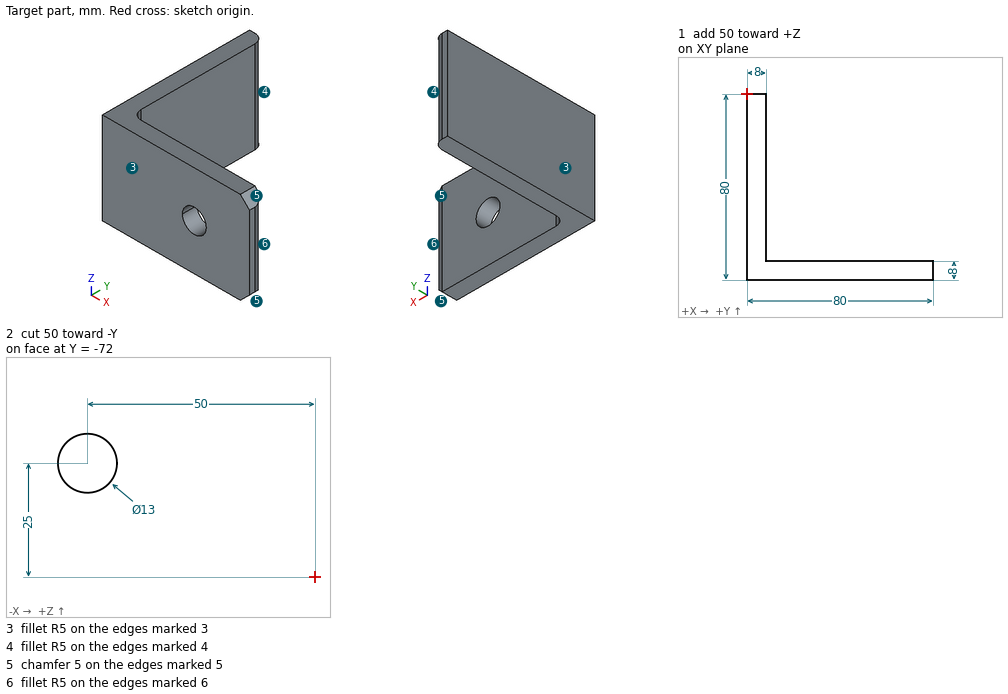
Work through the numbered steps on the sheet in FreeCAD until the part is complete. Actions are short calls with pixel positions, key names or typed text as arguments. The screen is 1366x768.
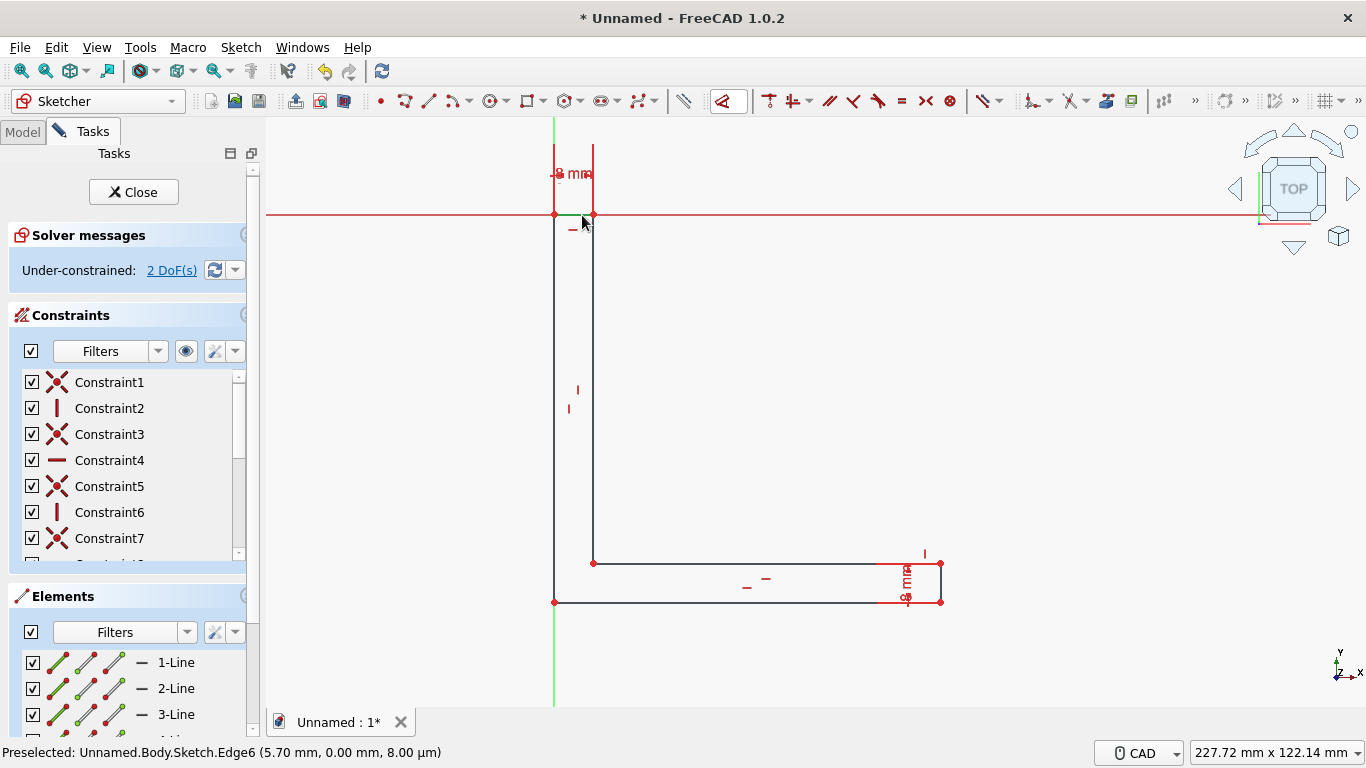
click(554, 331)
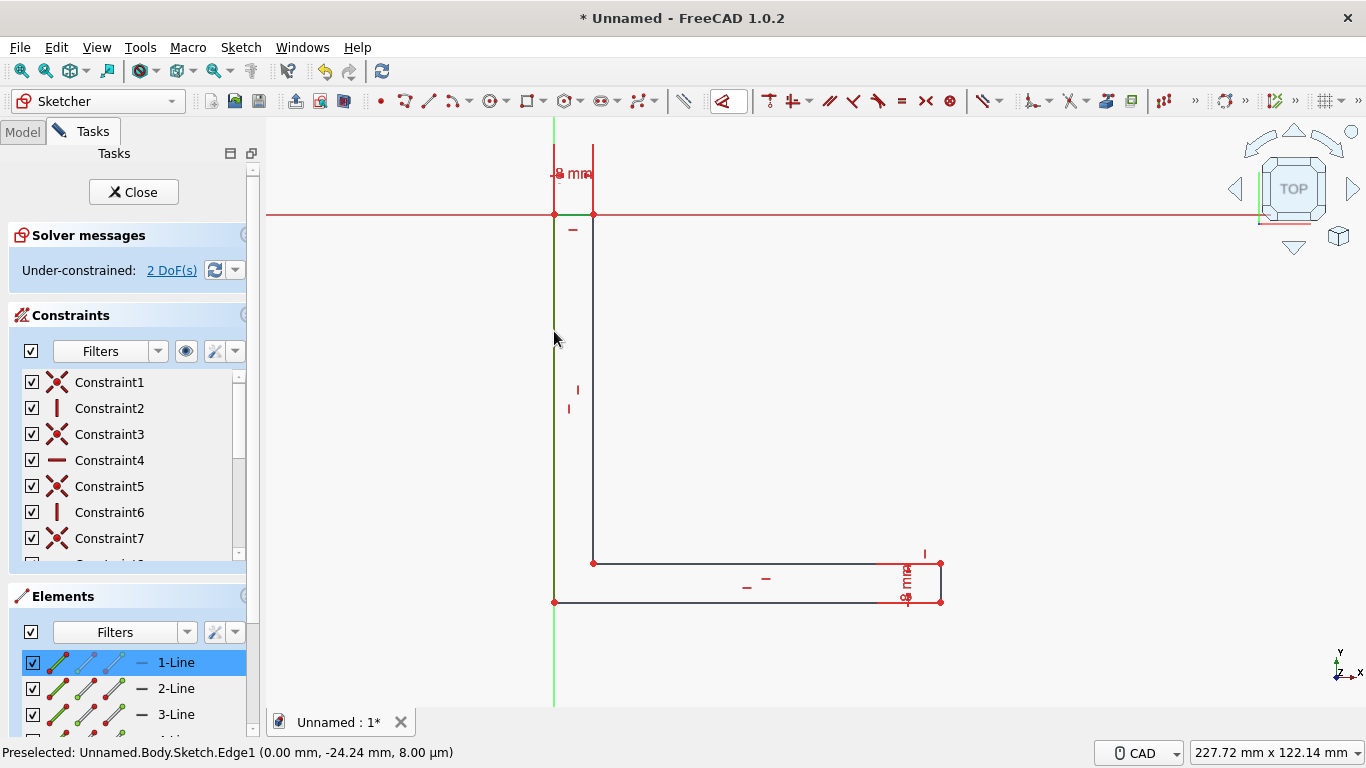
click(742, 102)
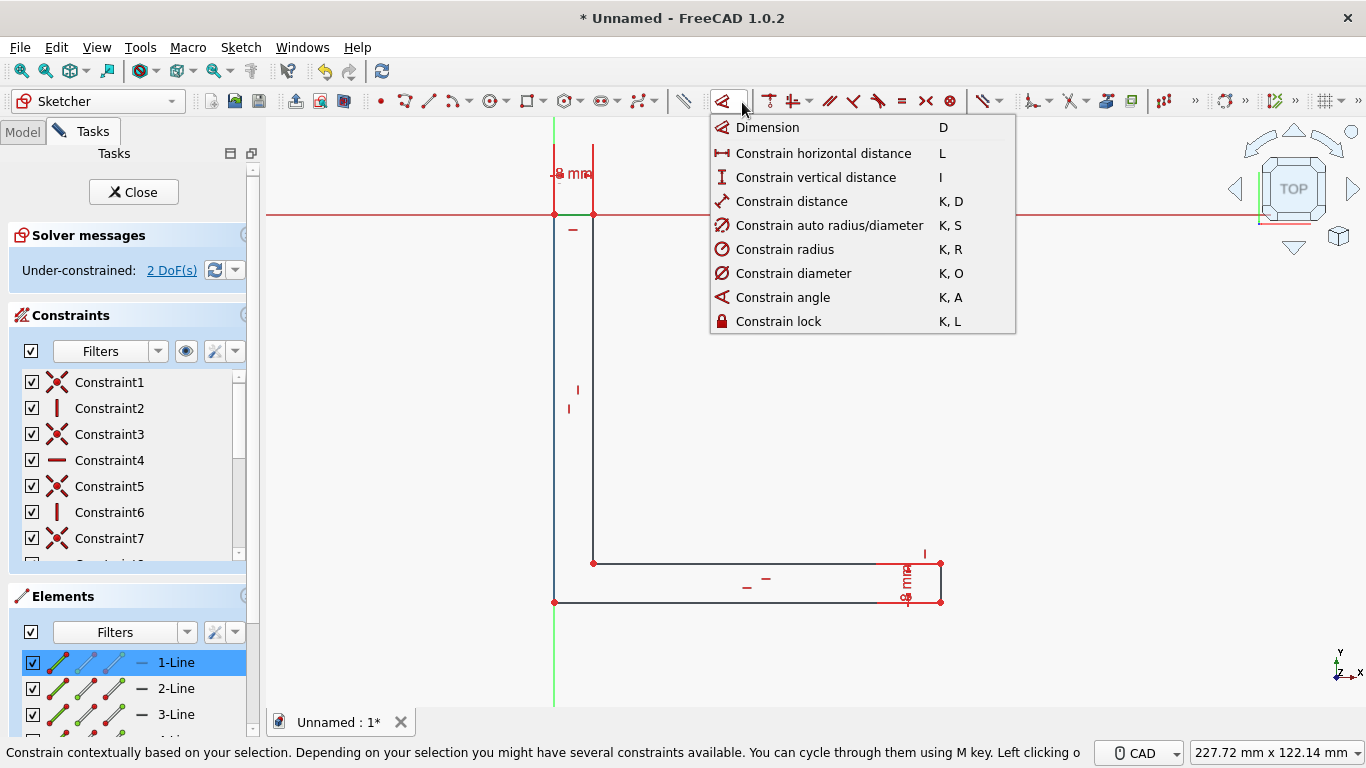
click(863, 177)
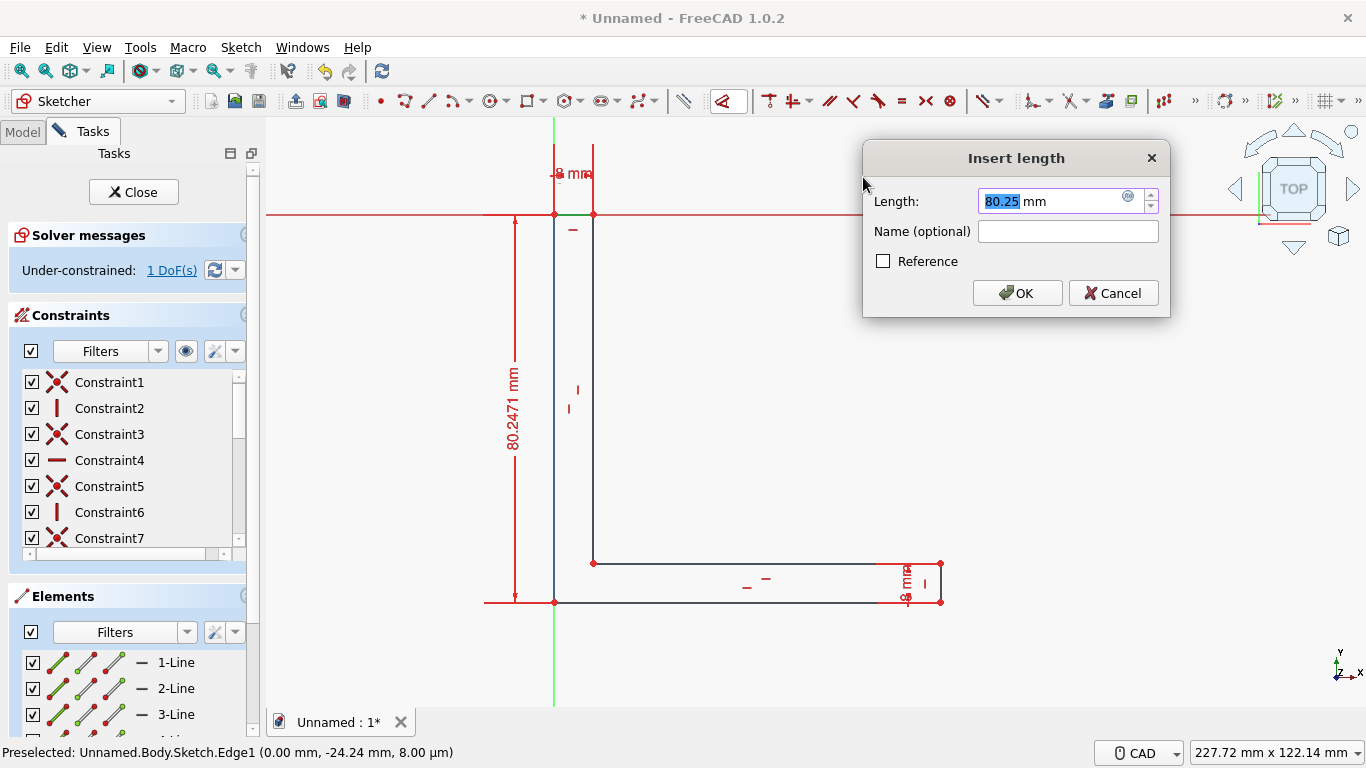
text(80)
key(Return)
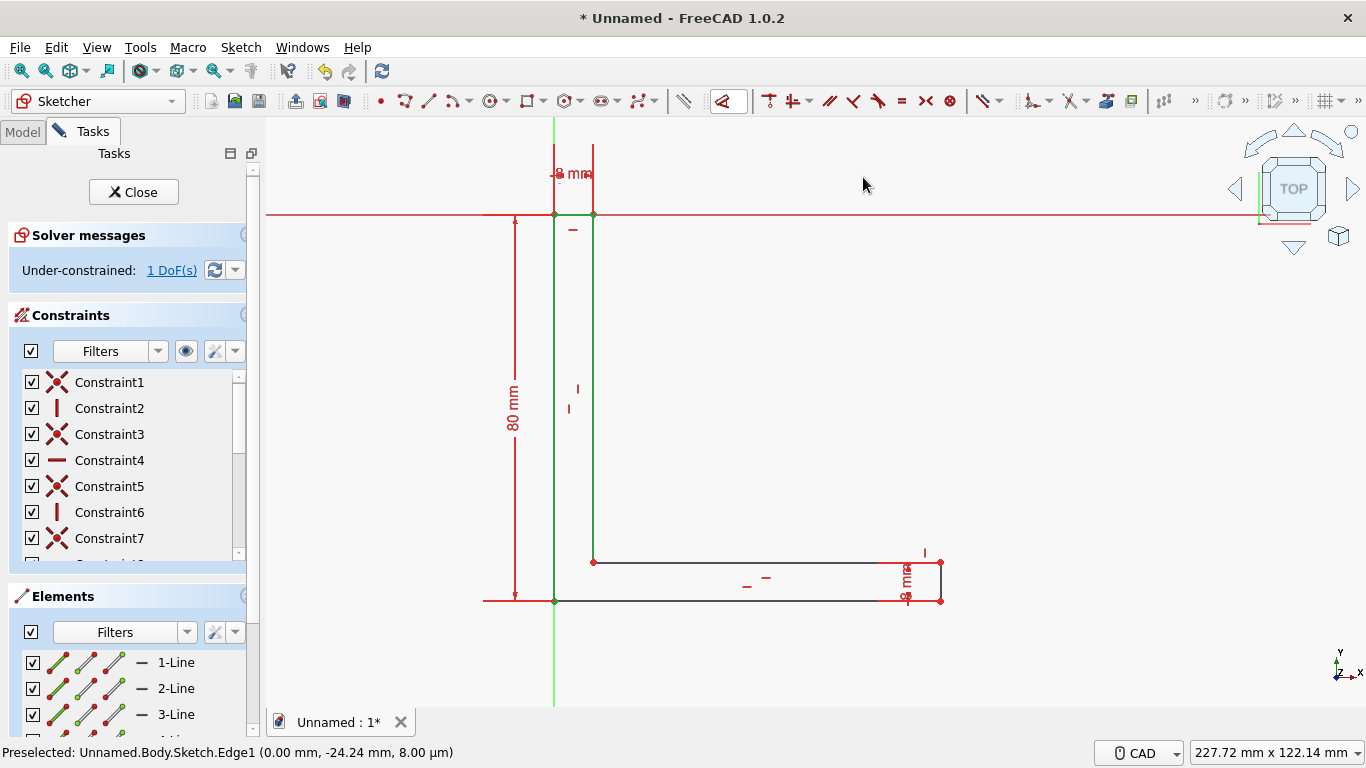
click(670, 601)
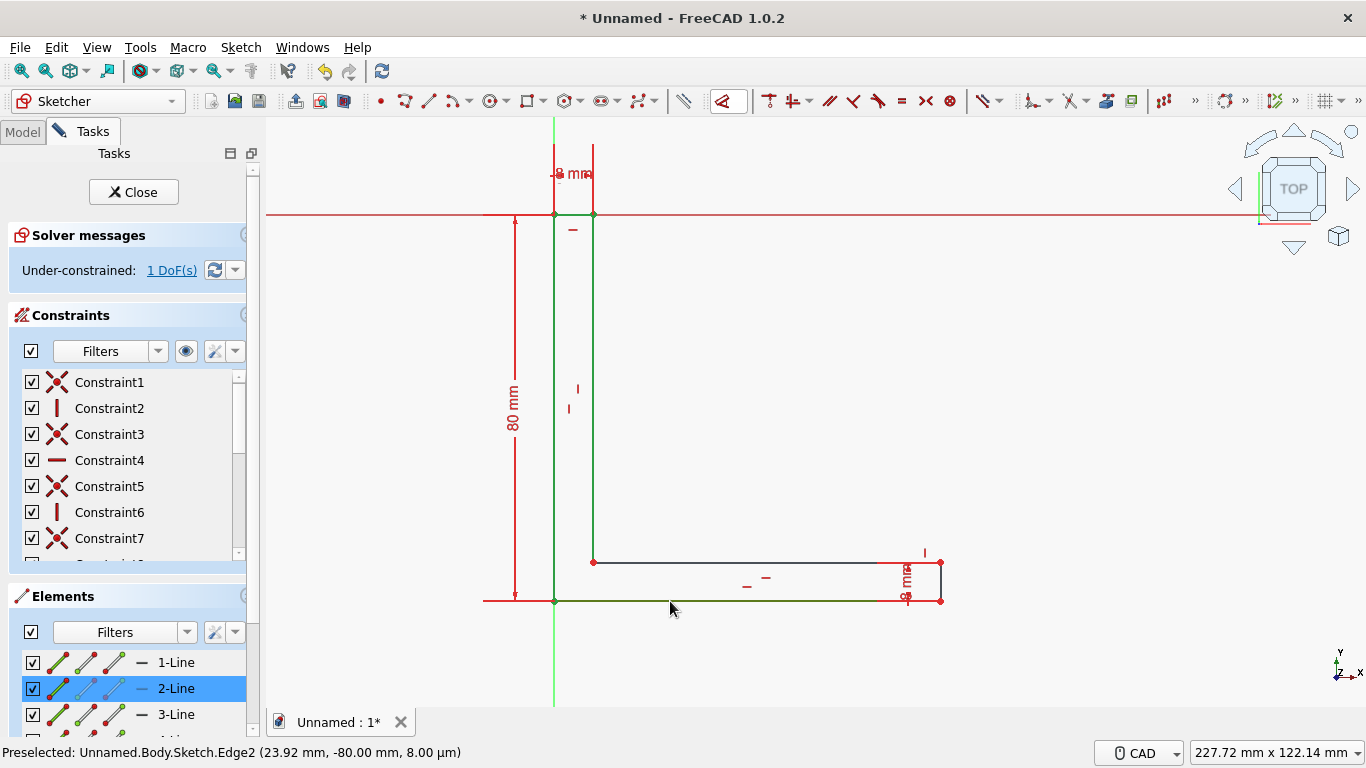
key(l)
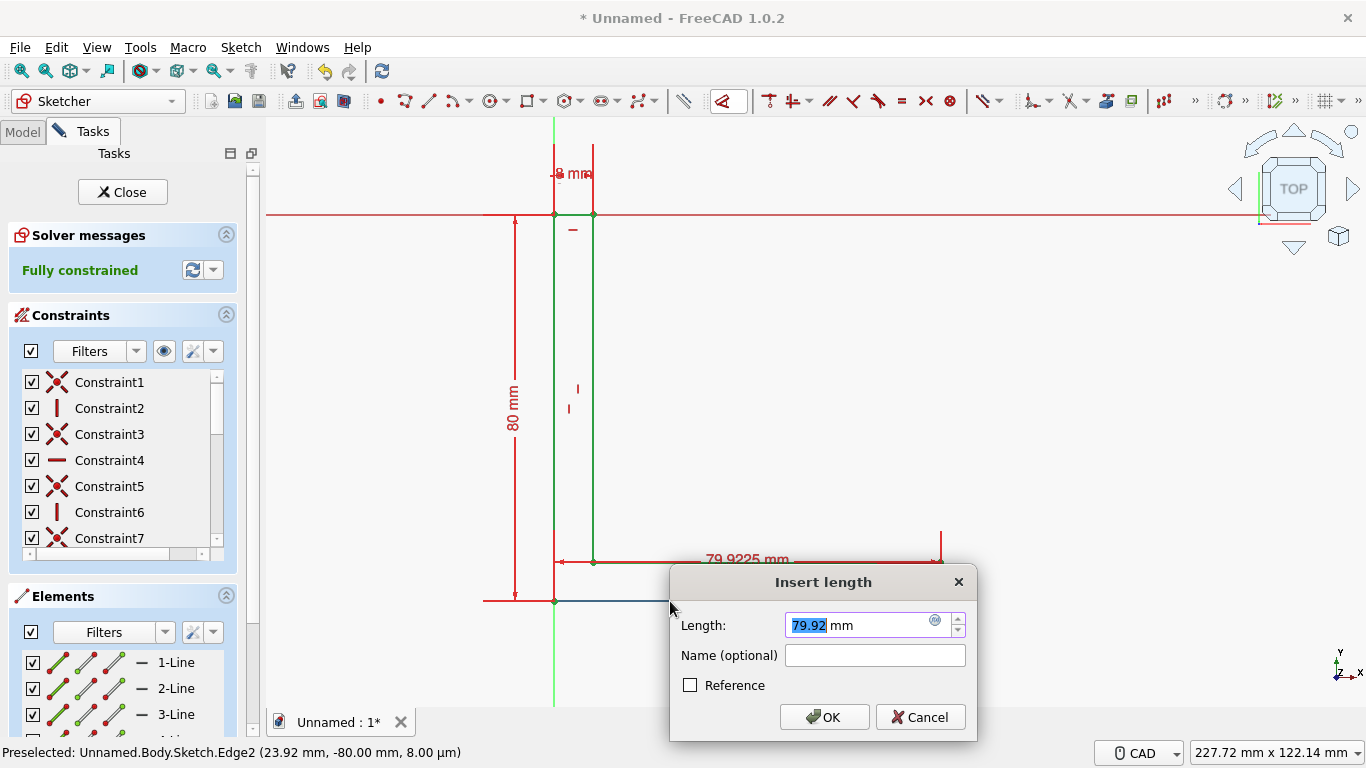
text(80)
key(Return)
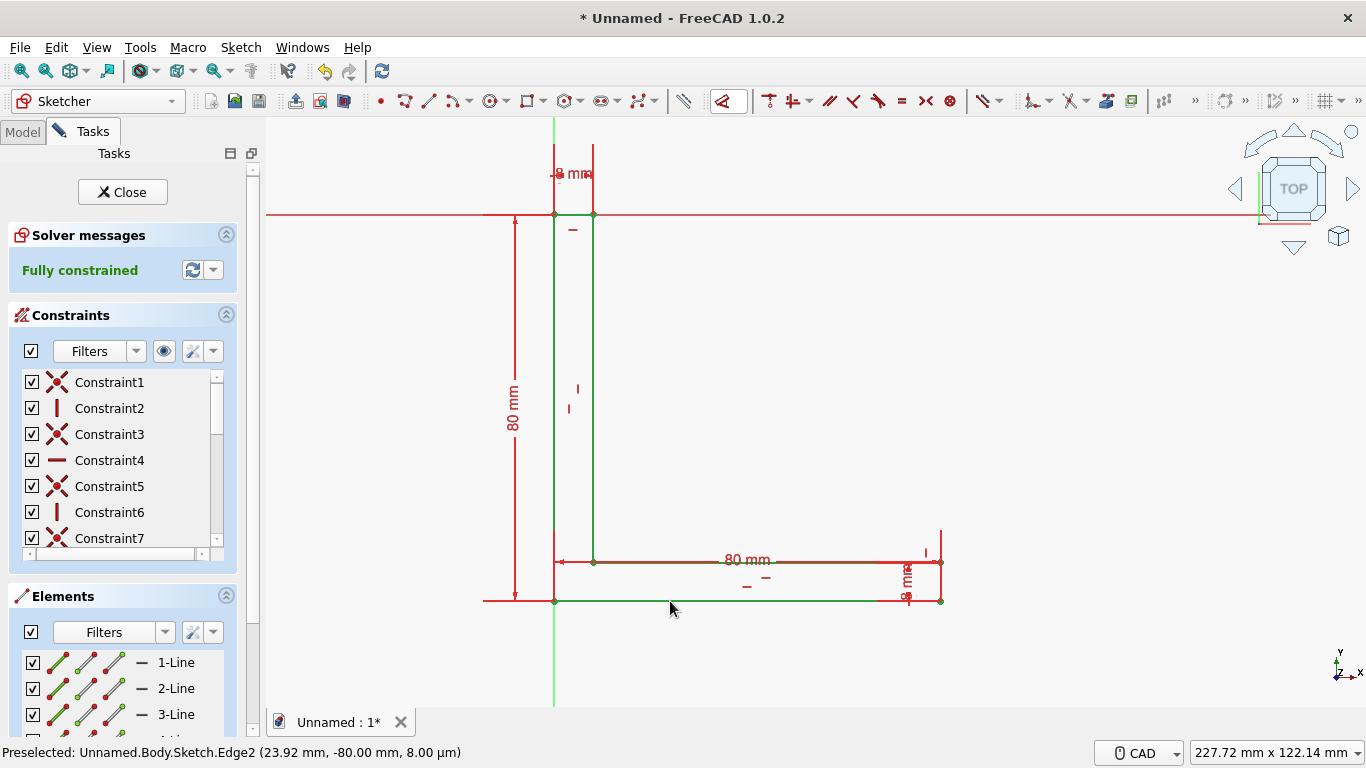
click(123, 192)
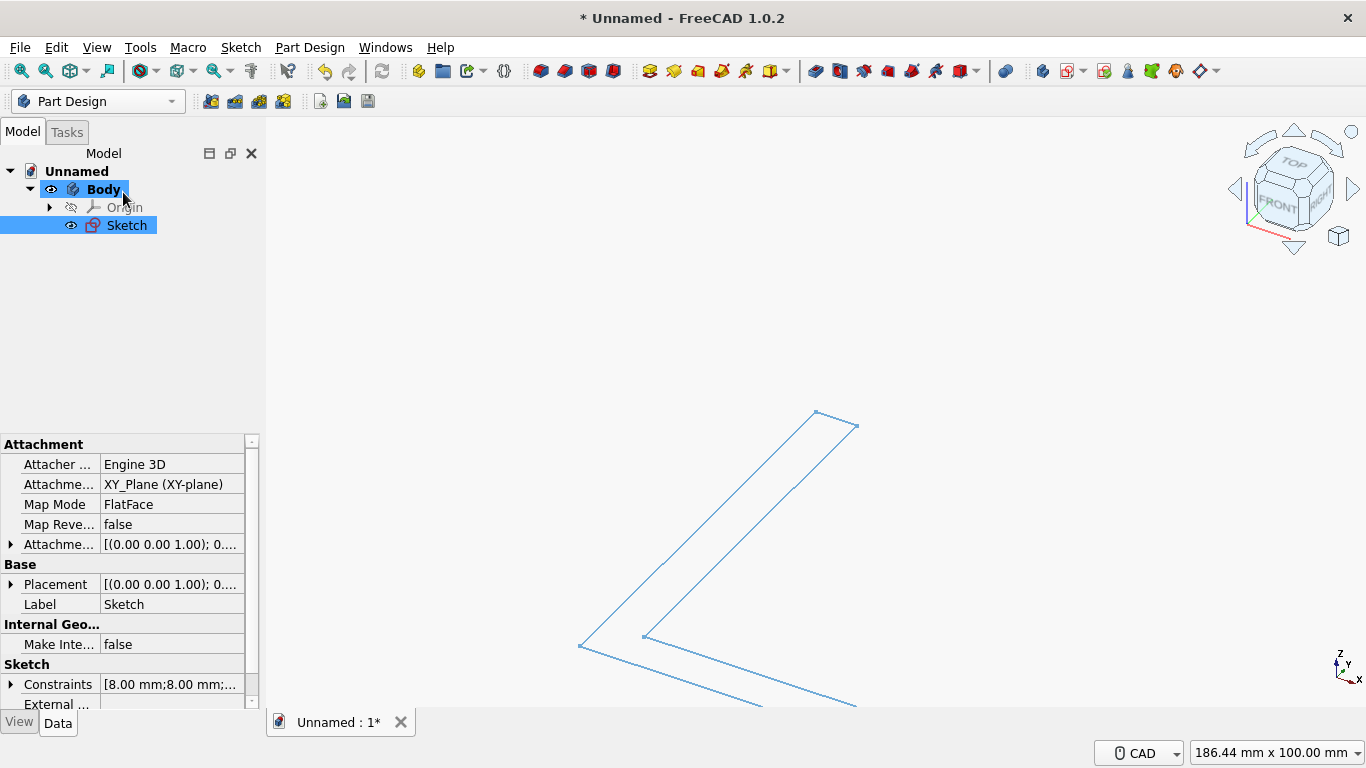
click(650, 72)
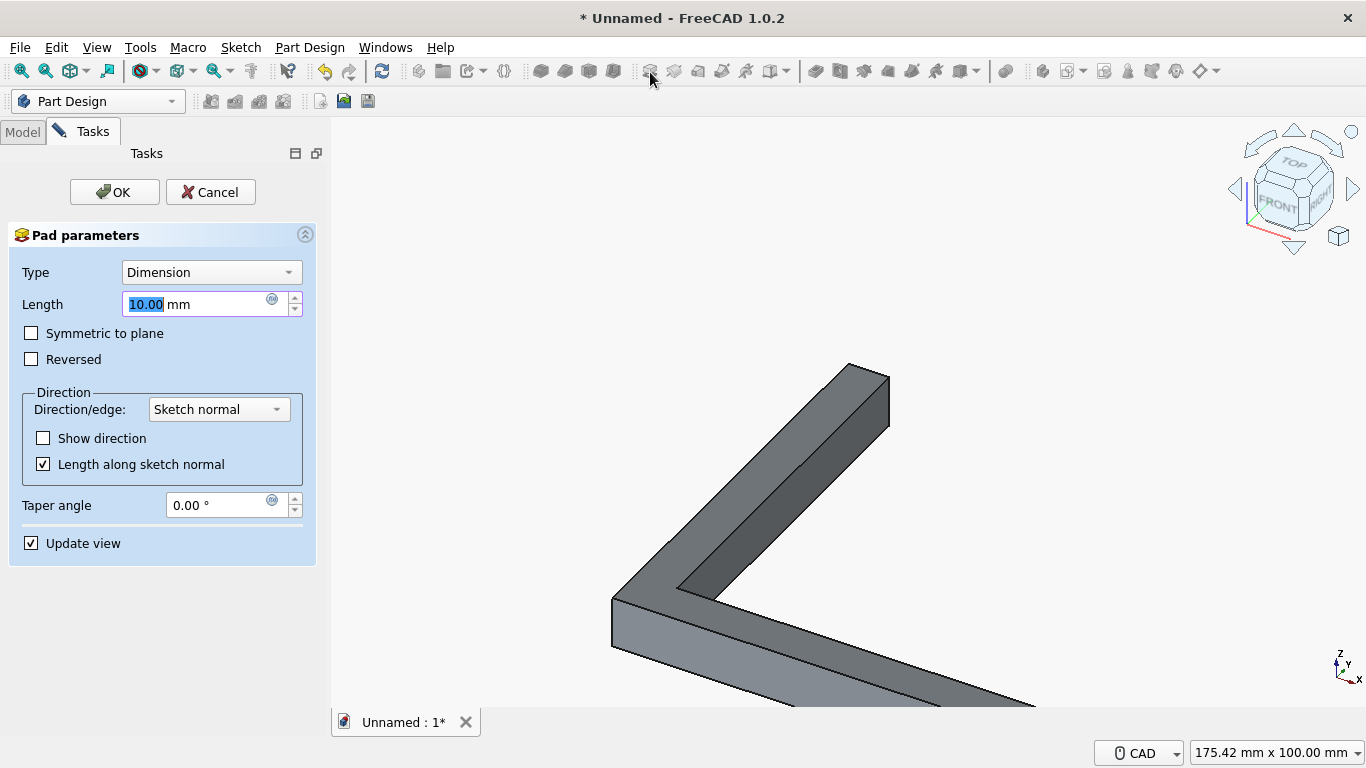
text(50)
key(Tab)